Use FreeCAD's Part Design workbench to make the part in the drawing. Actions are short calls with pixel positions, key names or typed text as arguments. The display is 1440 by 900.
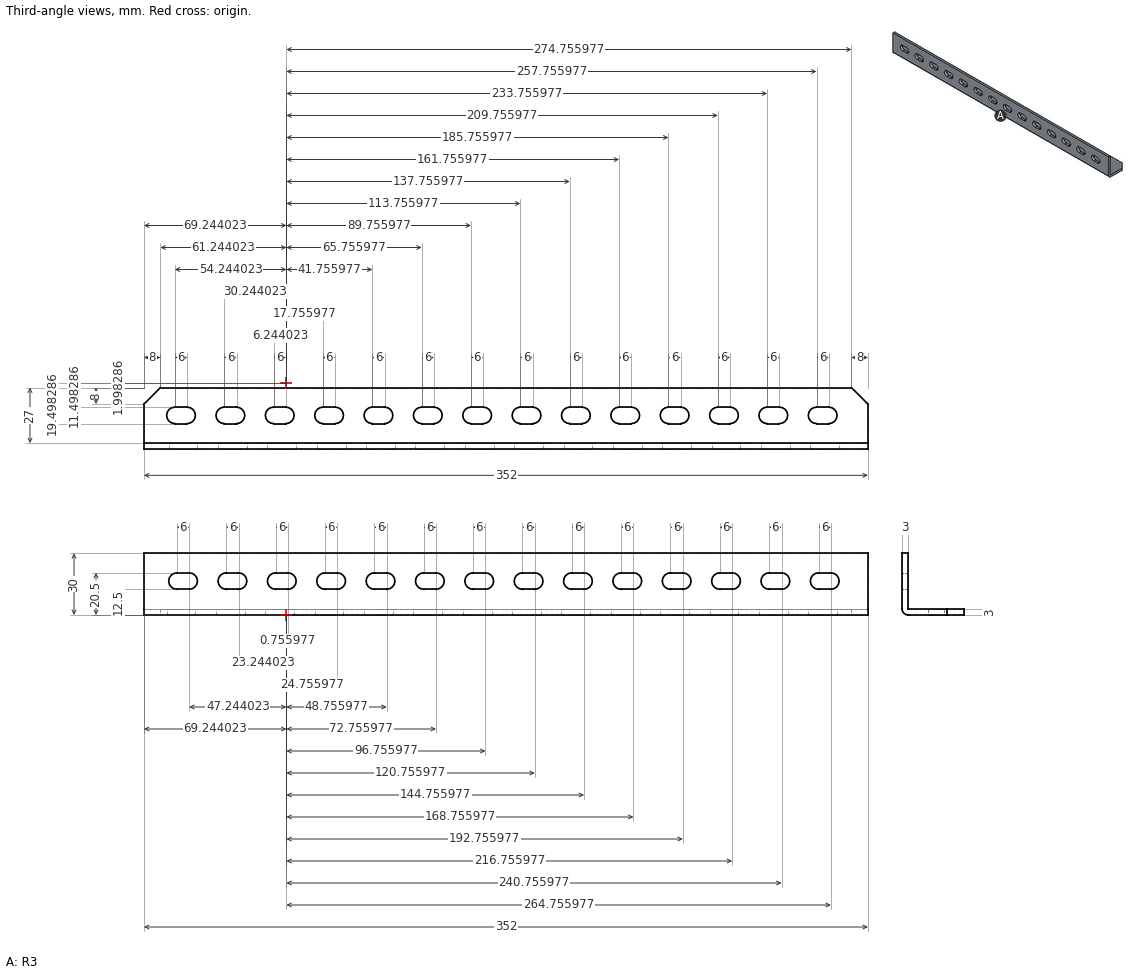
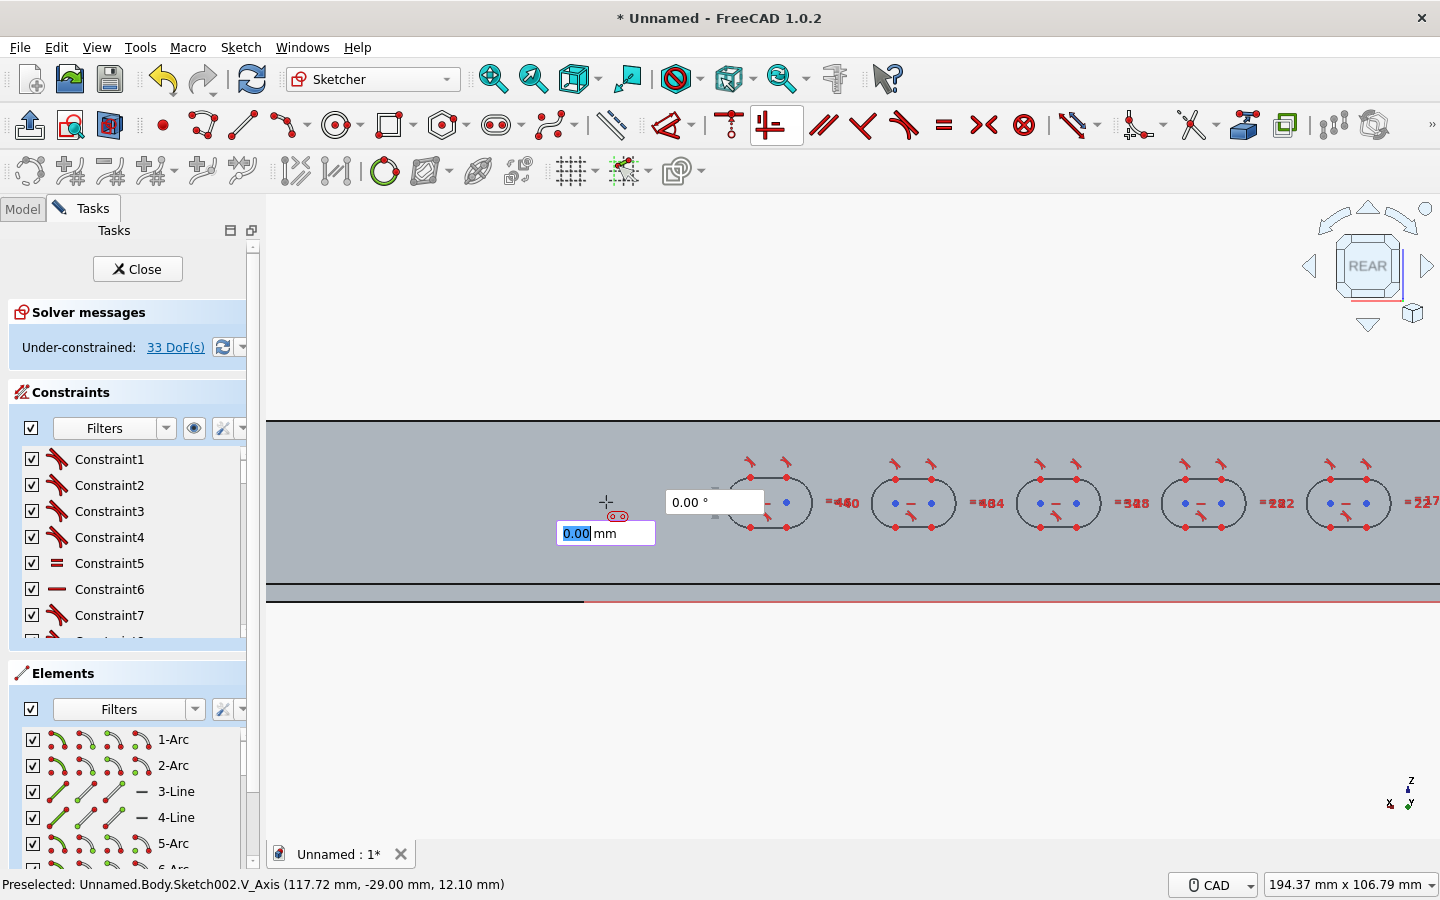
click(642, 502)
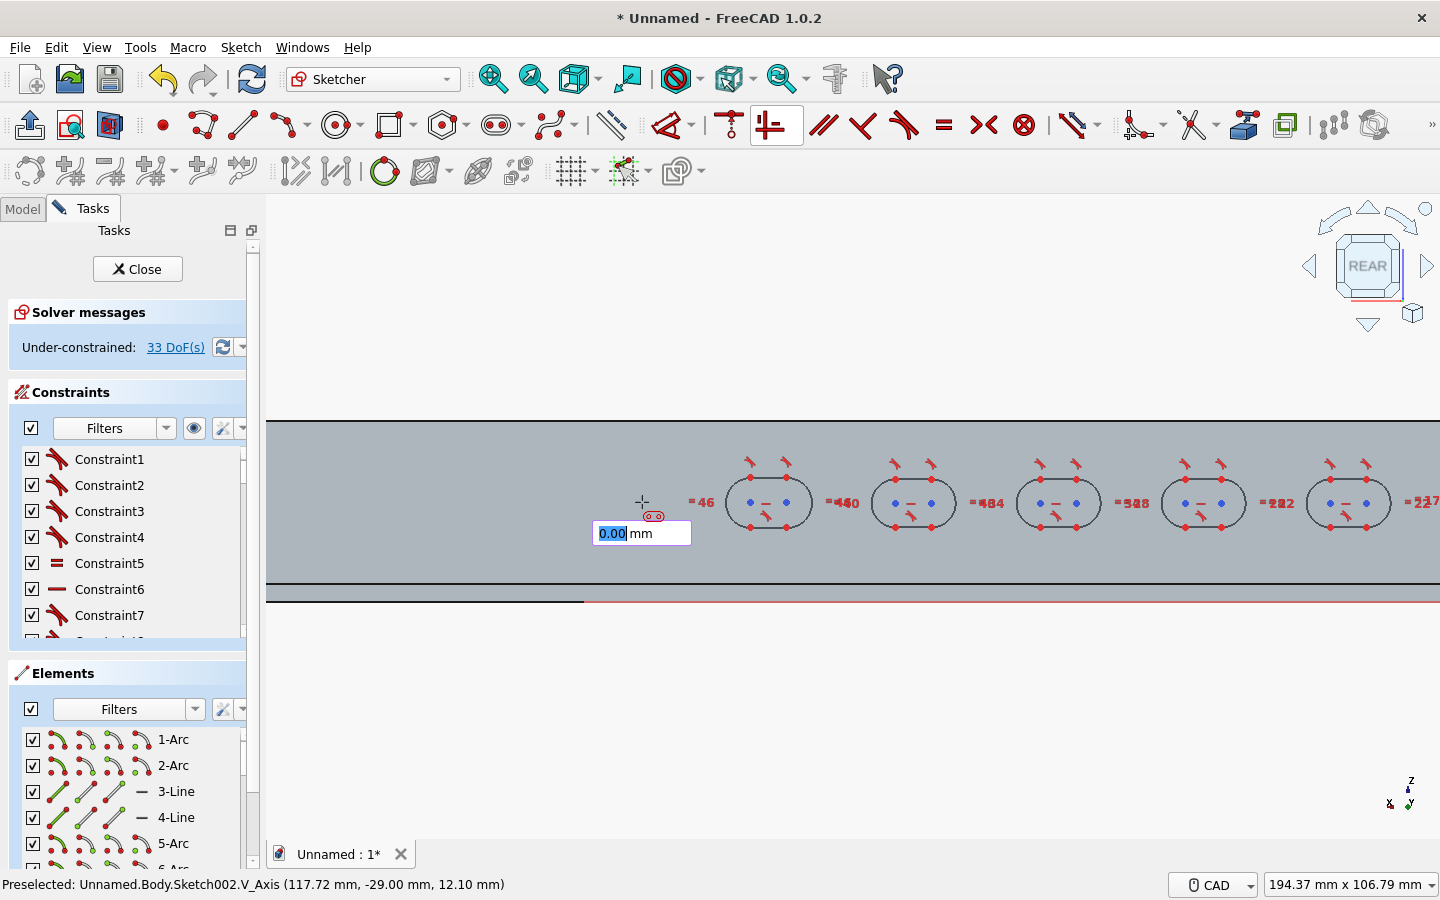
click(624, 527)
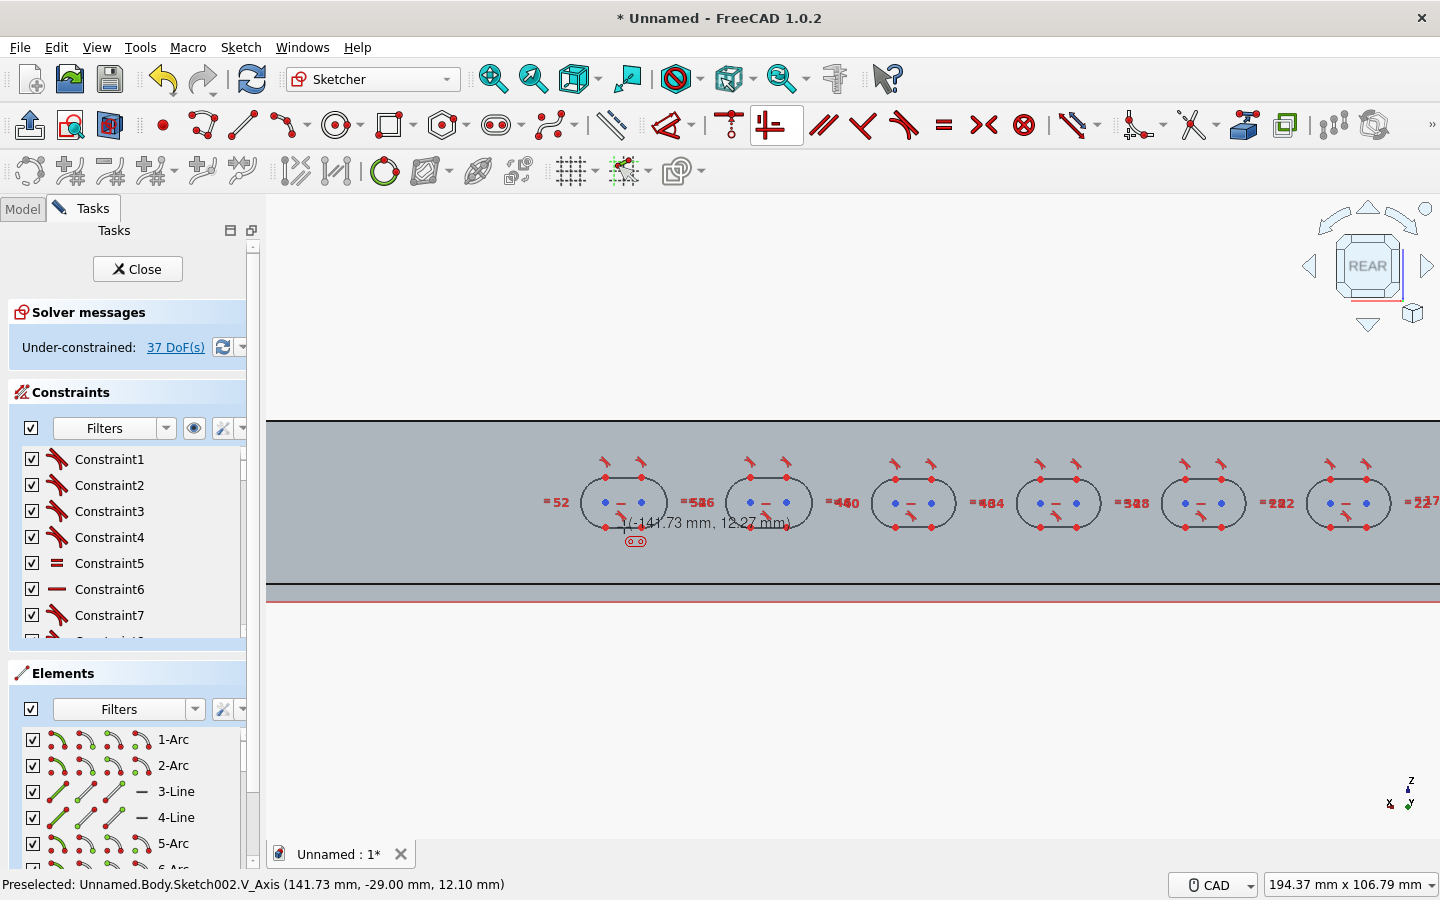
click(461, 502)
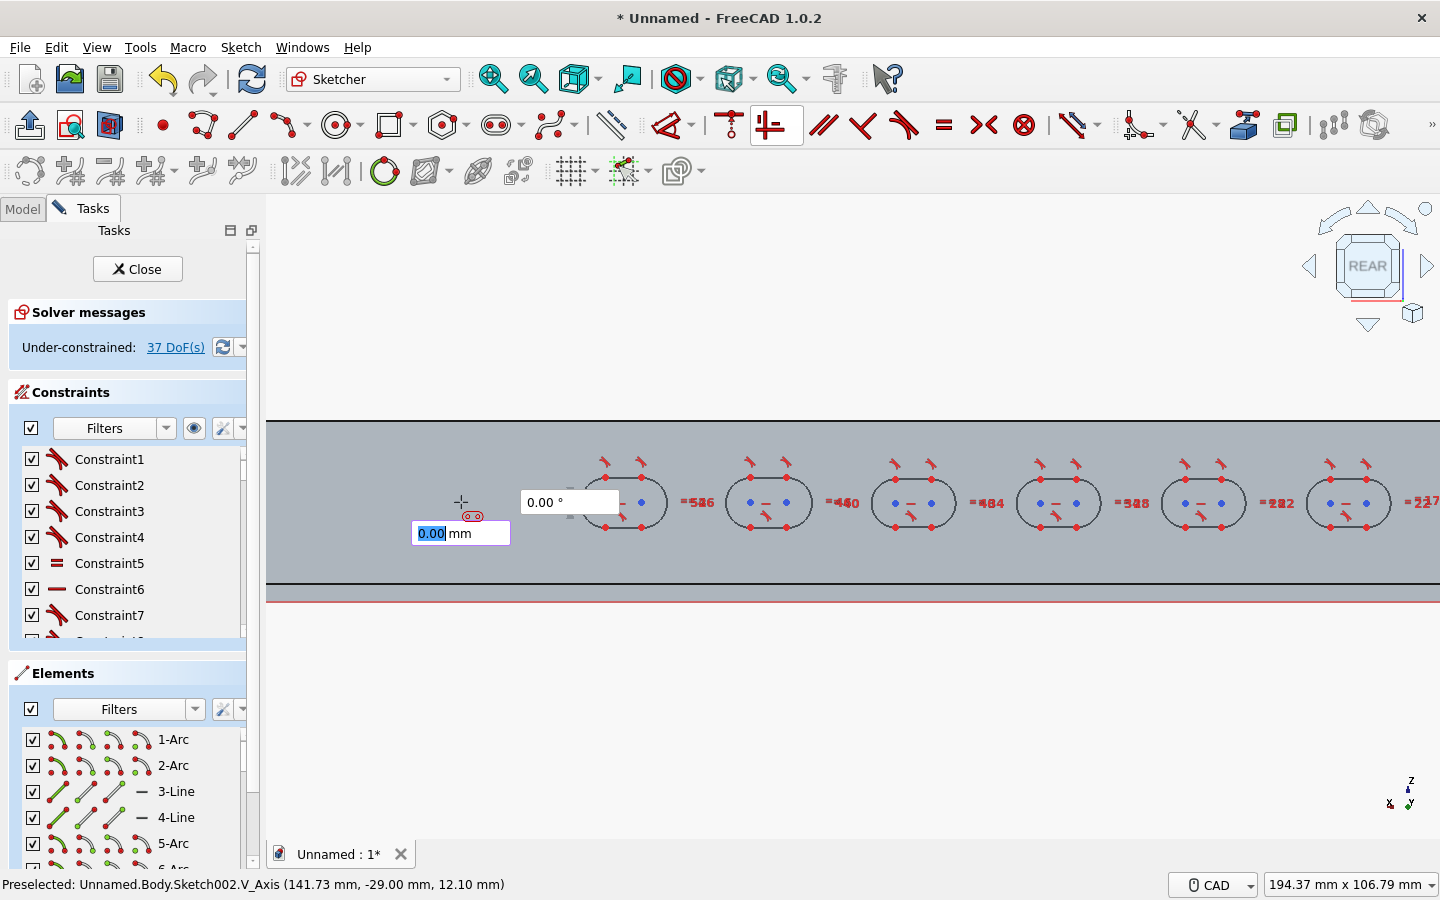
click(497, 502)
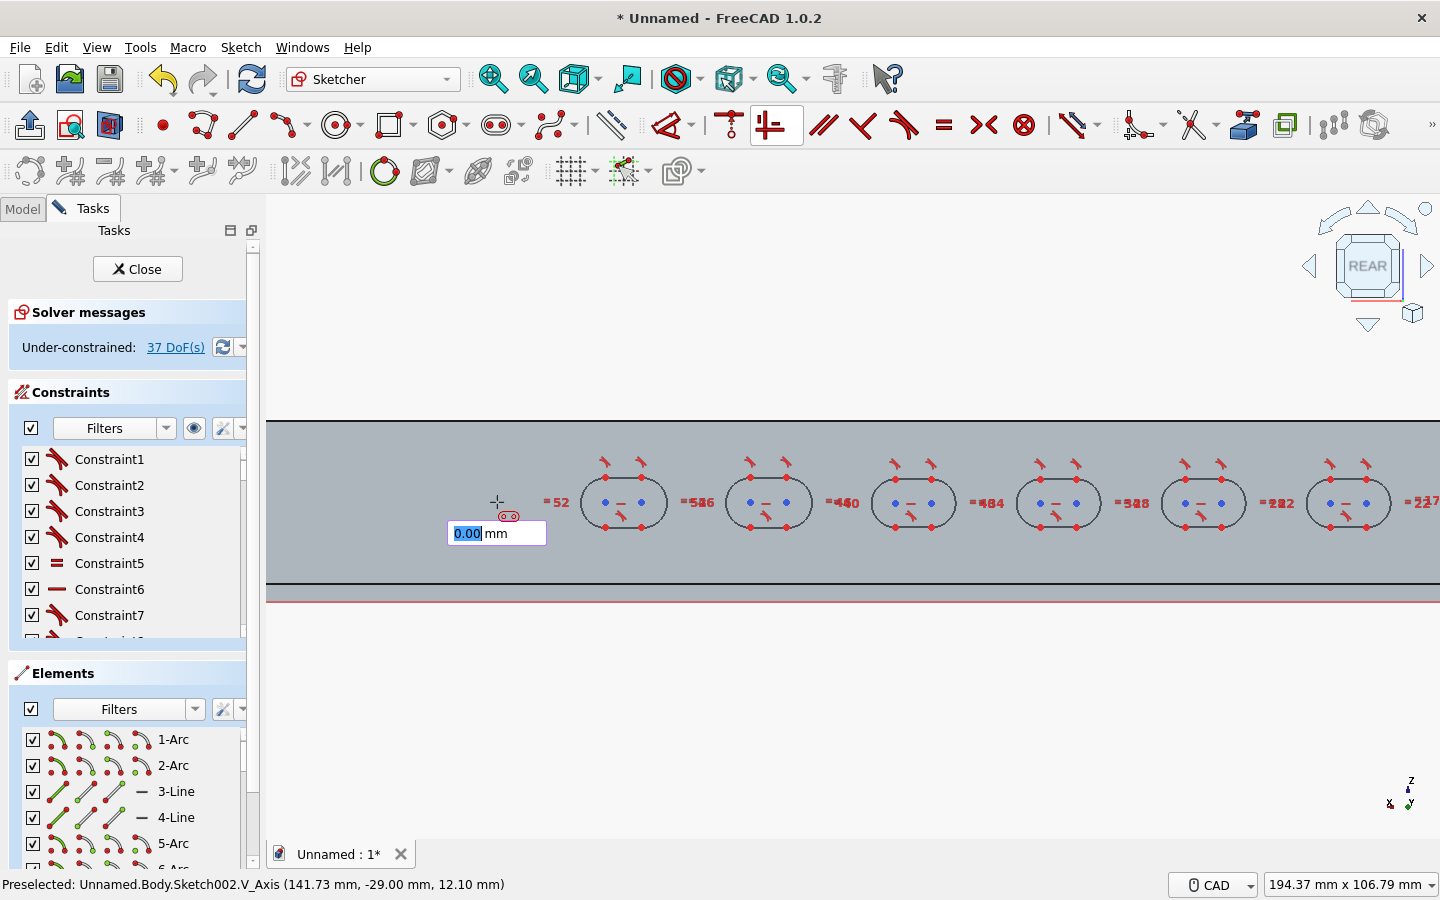
click(479, 527)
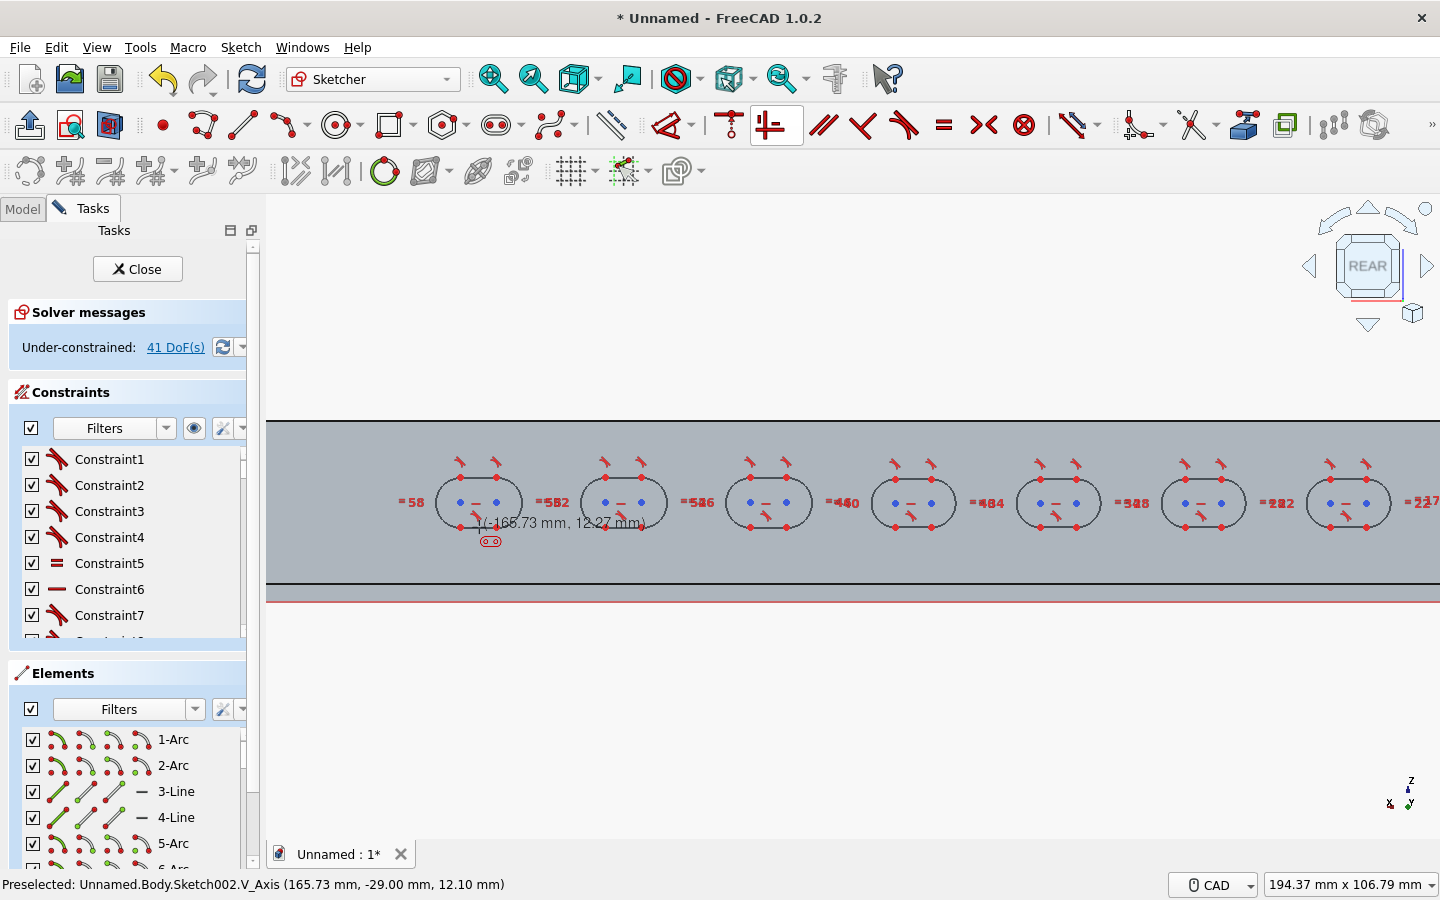
click(316, 502)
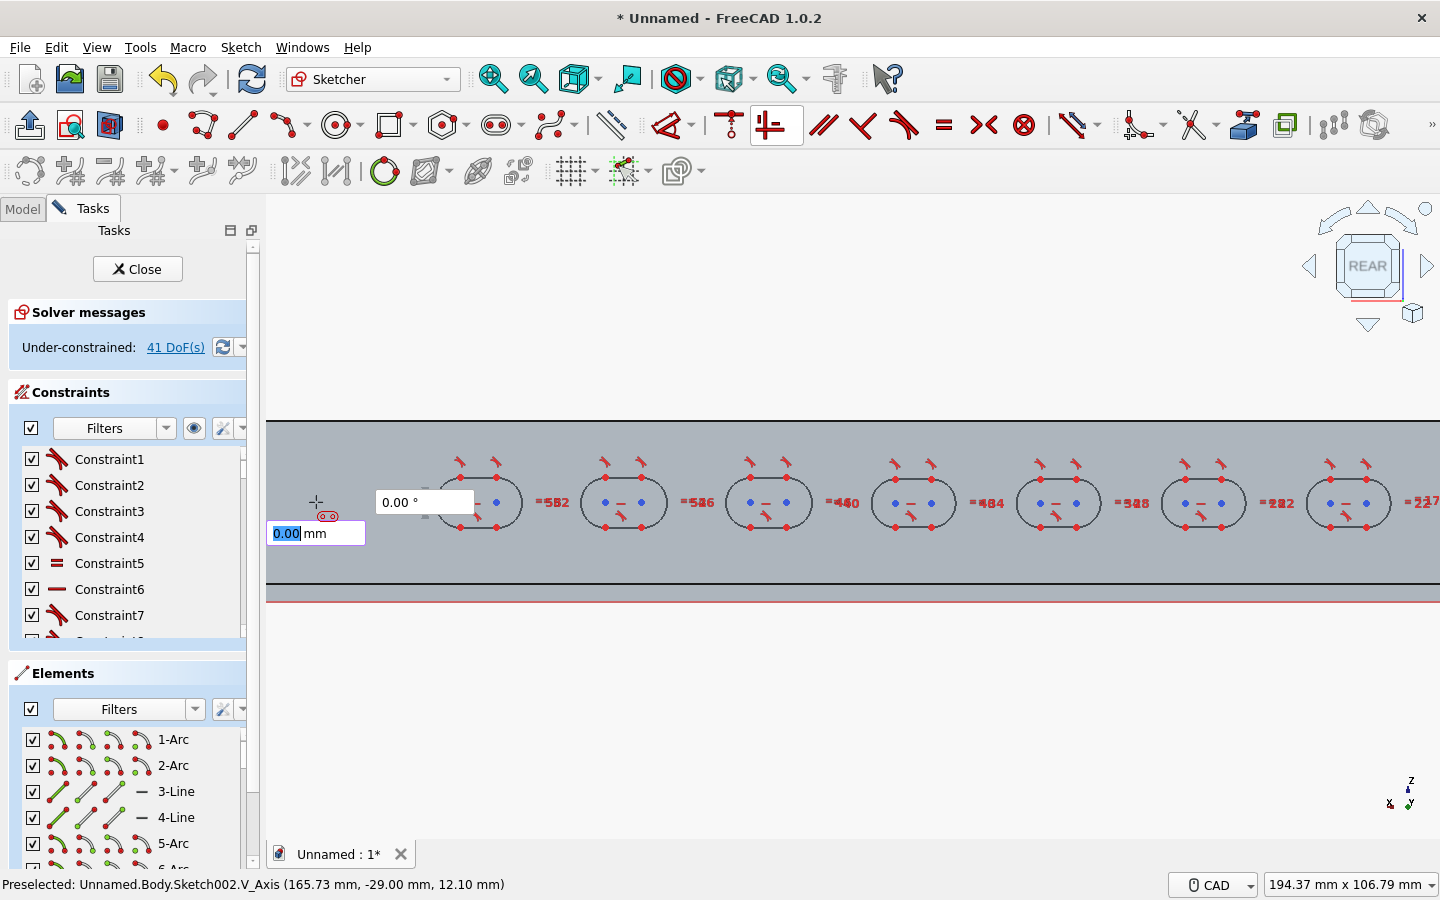
click(352, 502)